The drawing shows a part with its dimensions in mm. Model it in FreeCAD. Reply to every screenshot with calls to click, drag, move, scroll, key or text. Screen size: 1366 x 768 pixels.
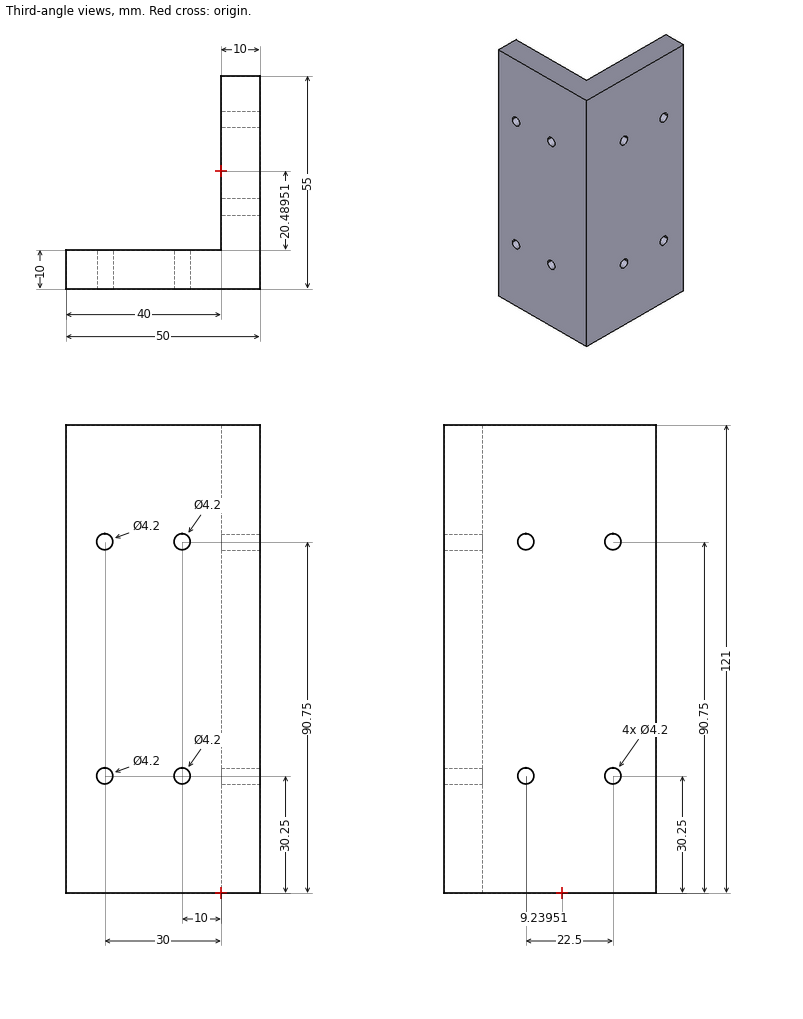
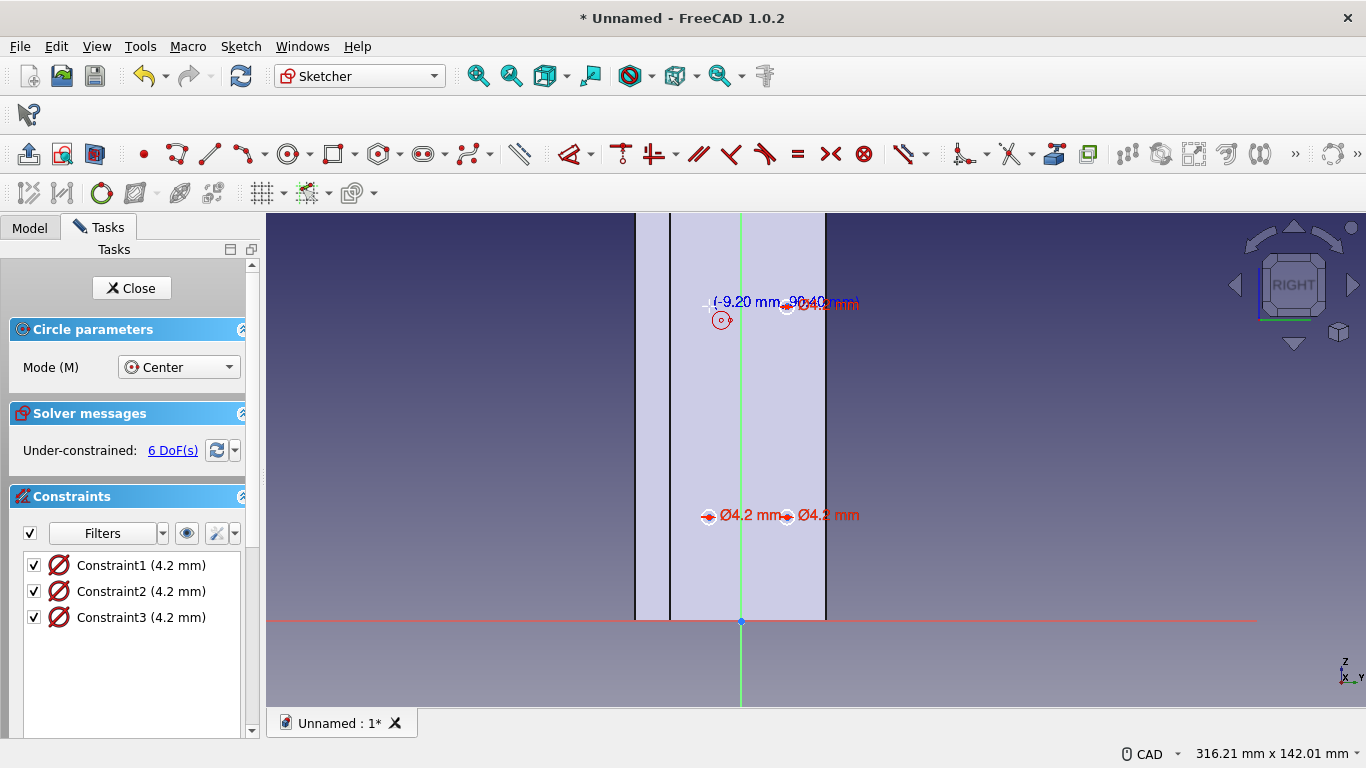
click(709, 306)
move(714, 301)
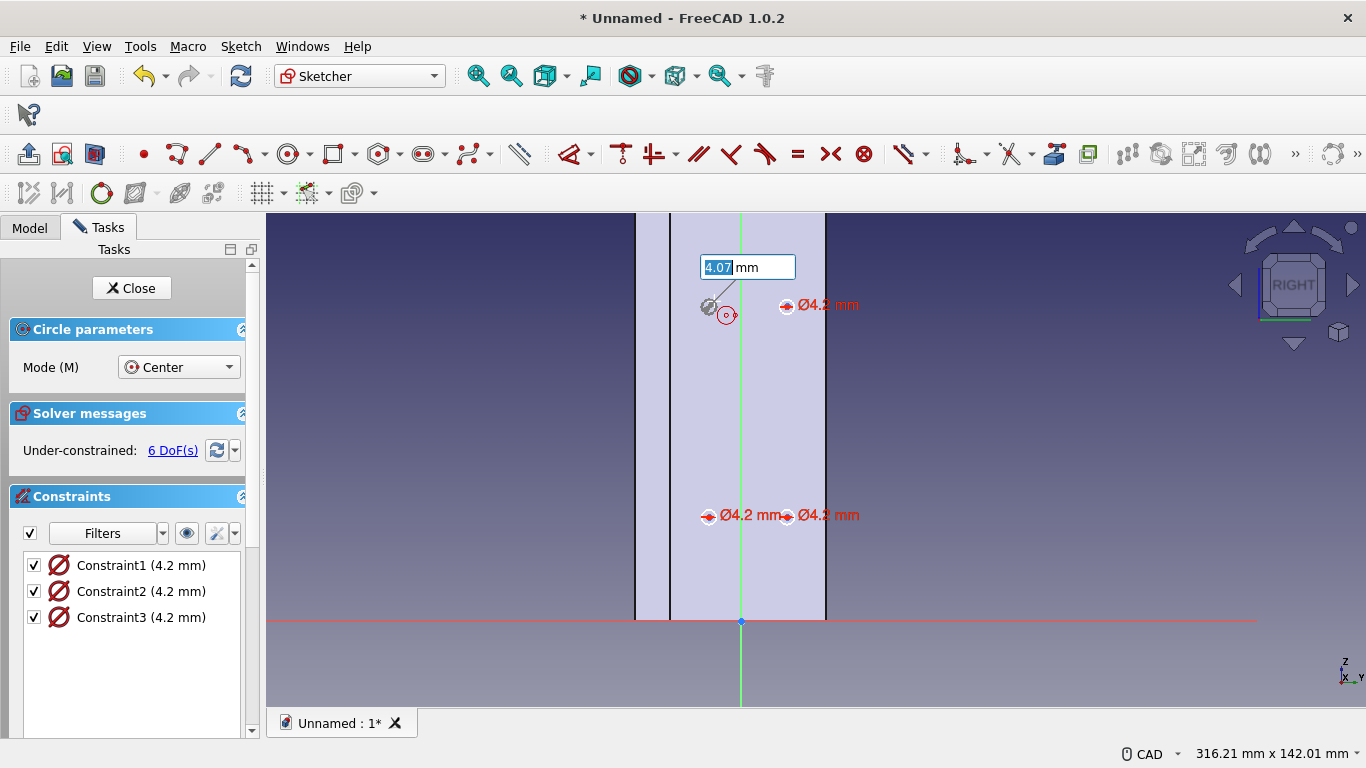
text(4.2)
key(Return)
key(Escape)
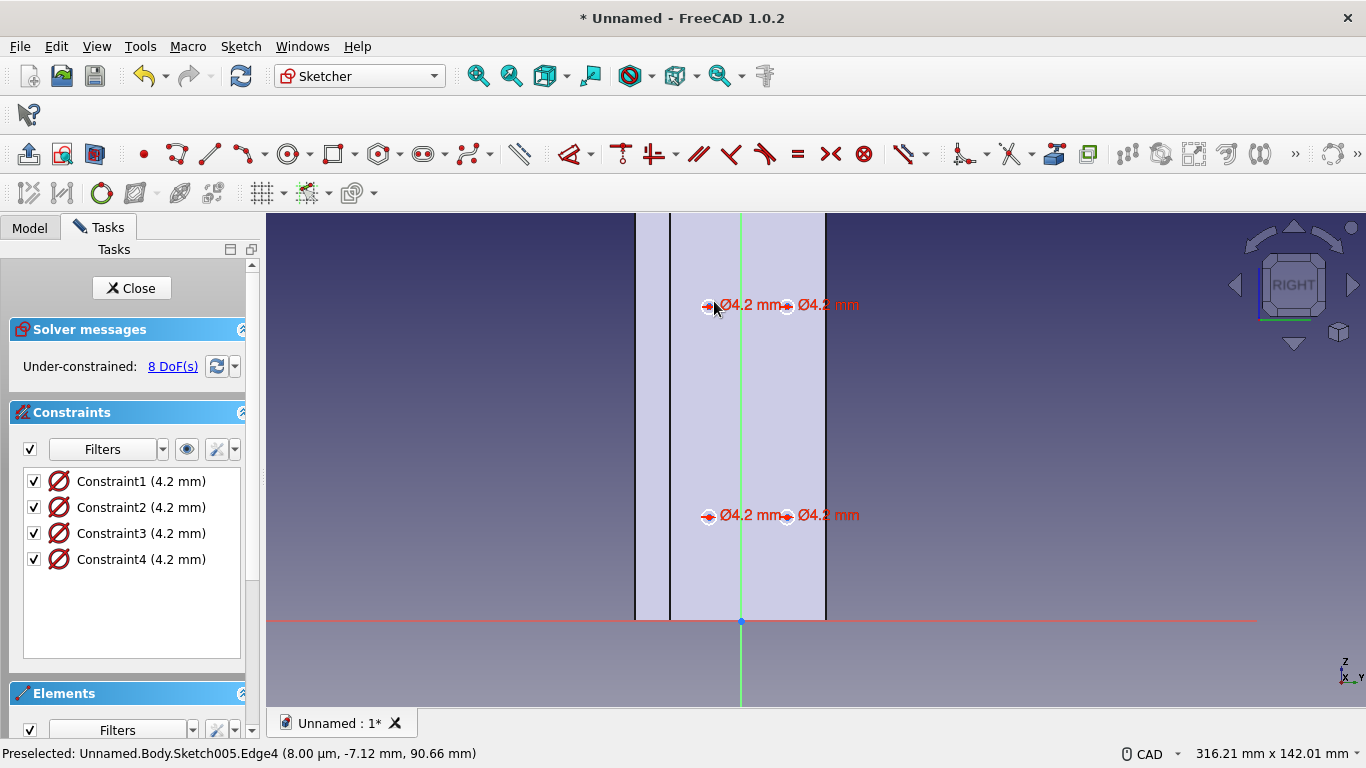
click(787, 517)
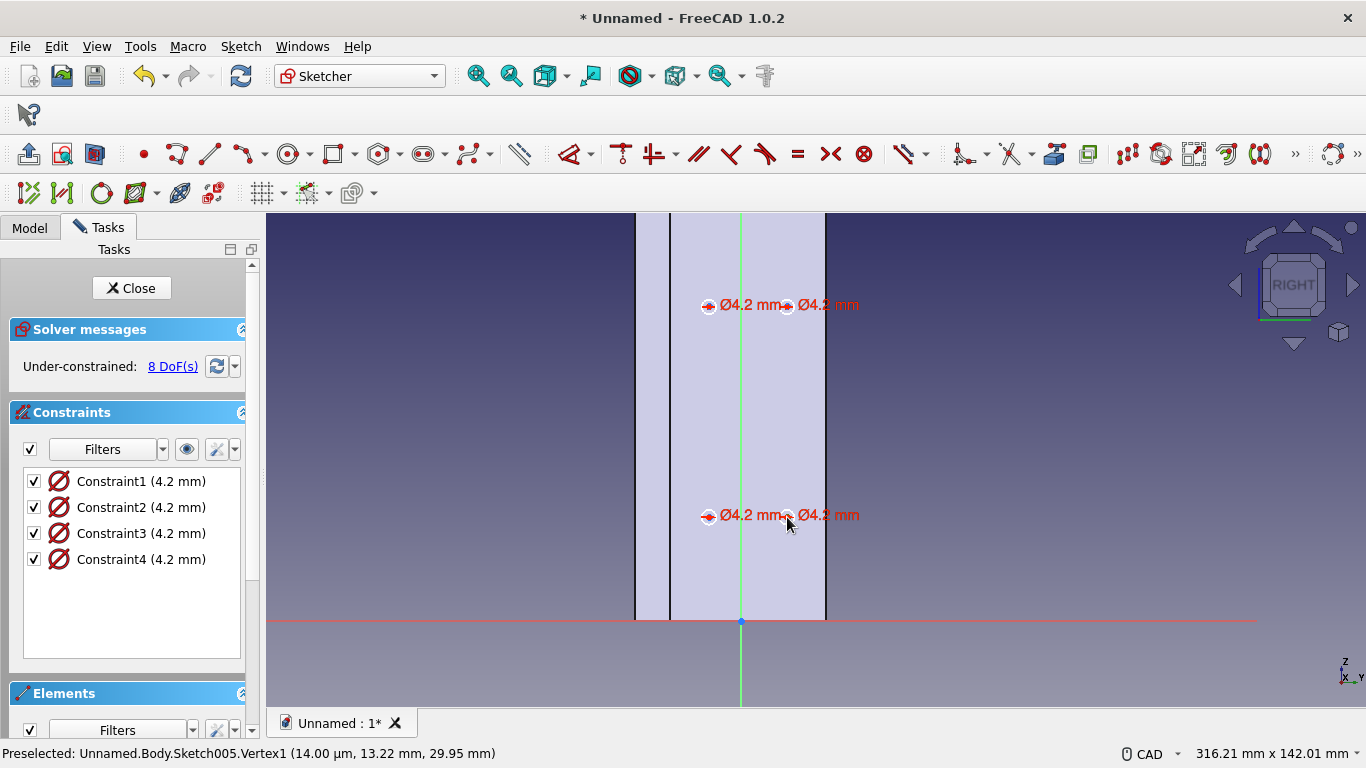
click(709, 517)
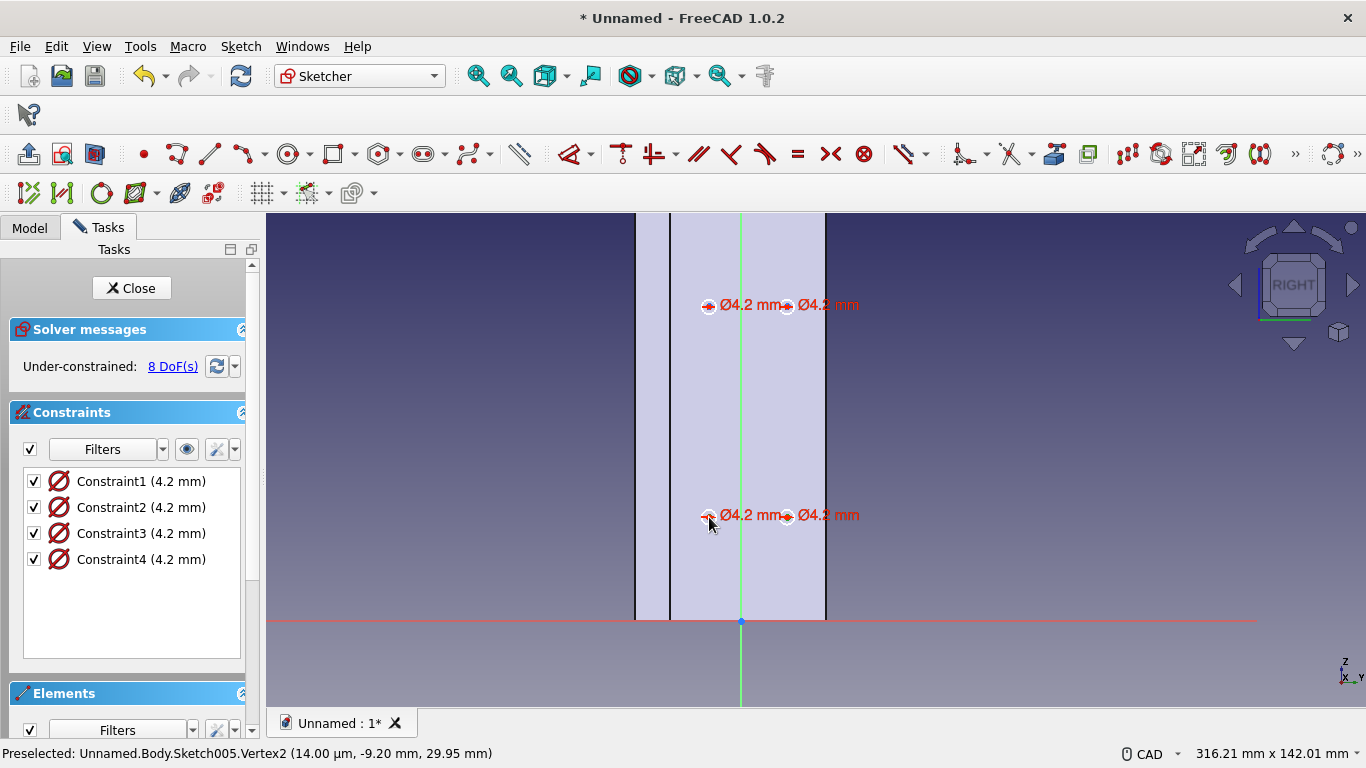
key(h)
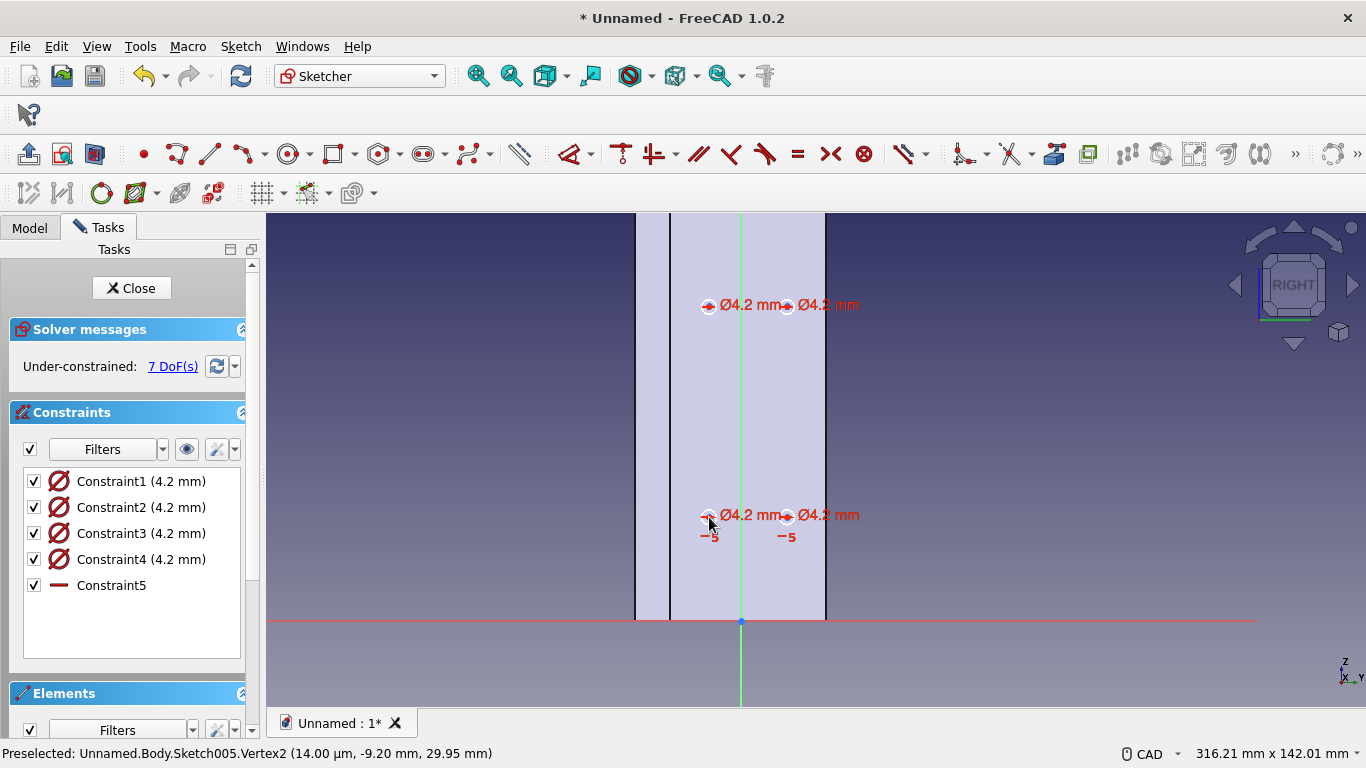
click(787, 517)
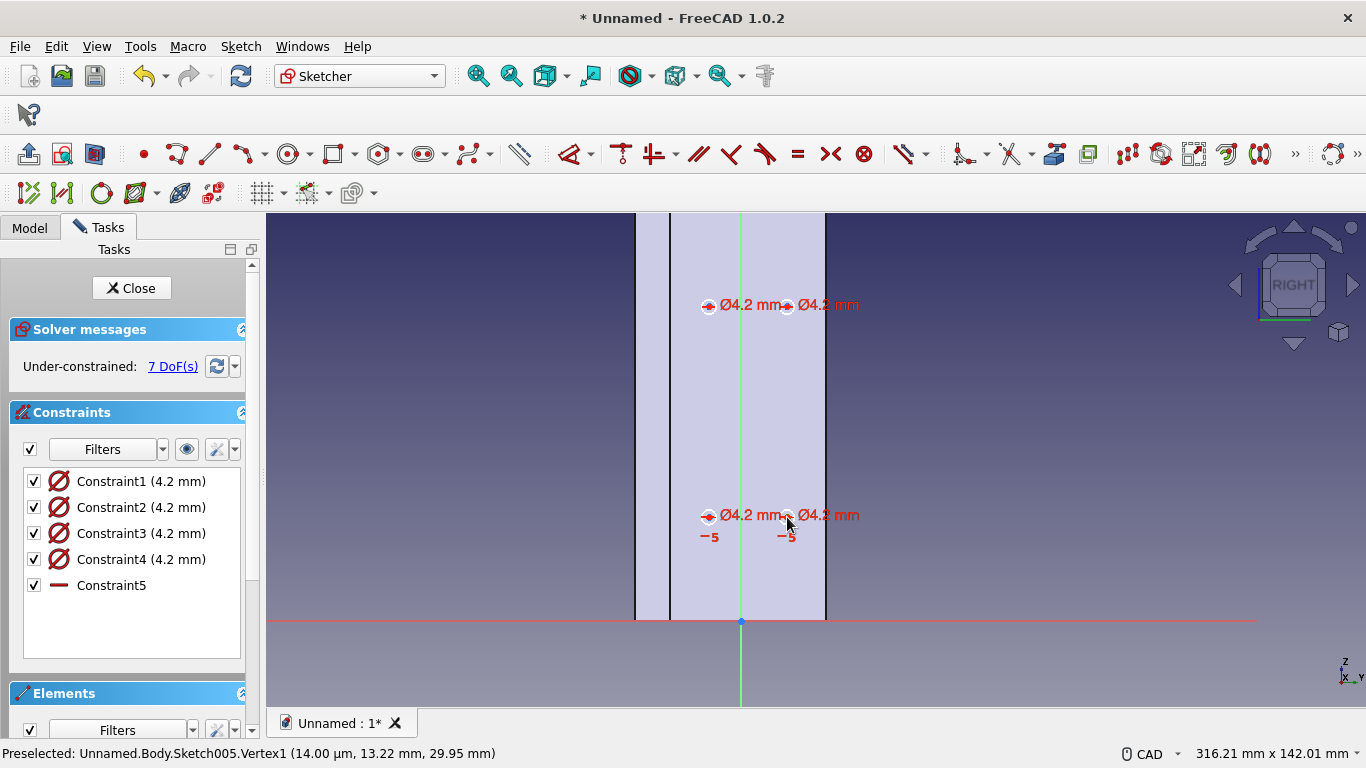
click(787, 307)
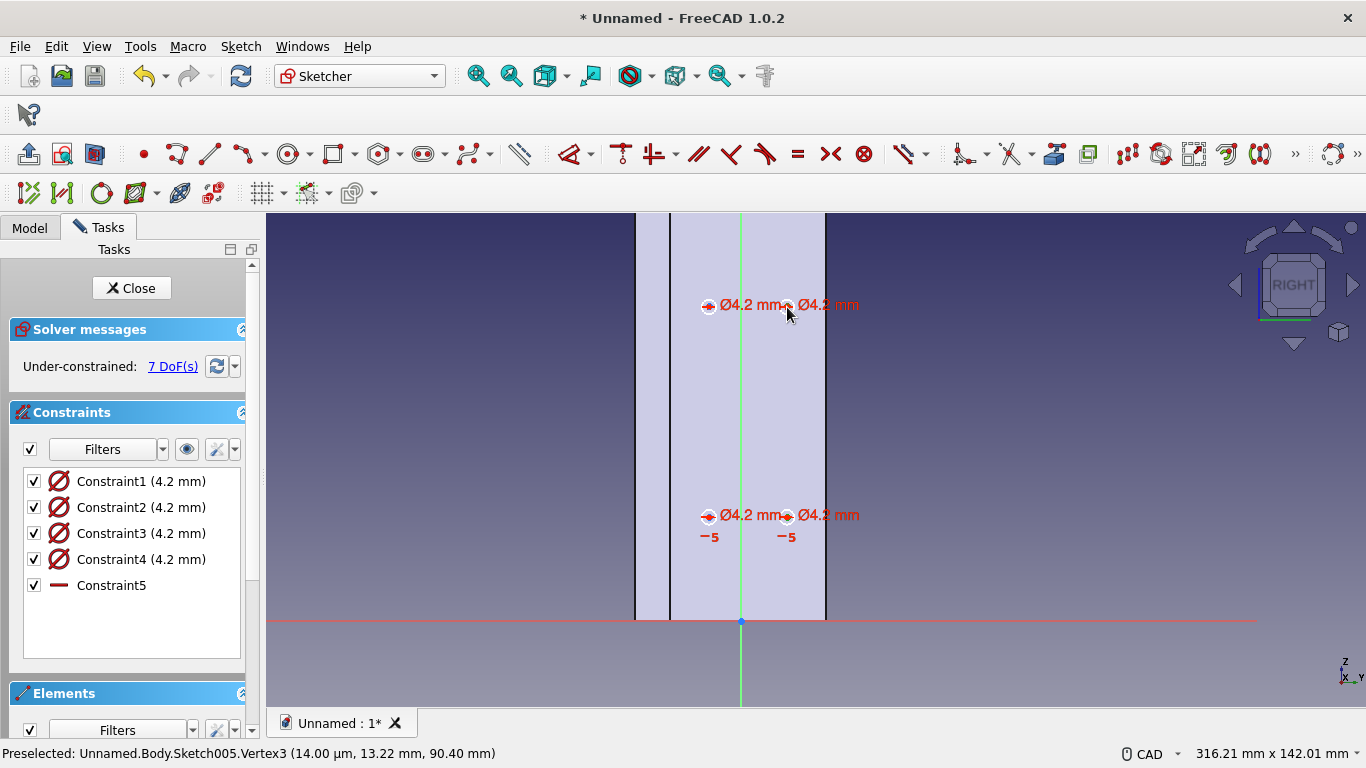
key(v)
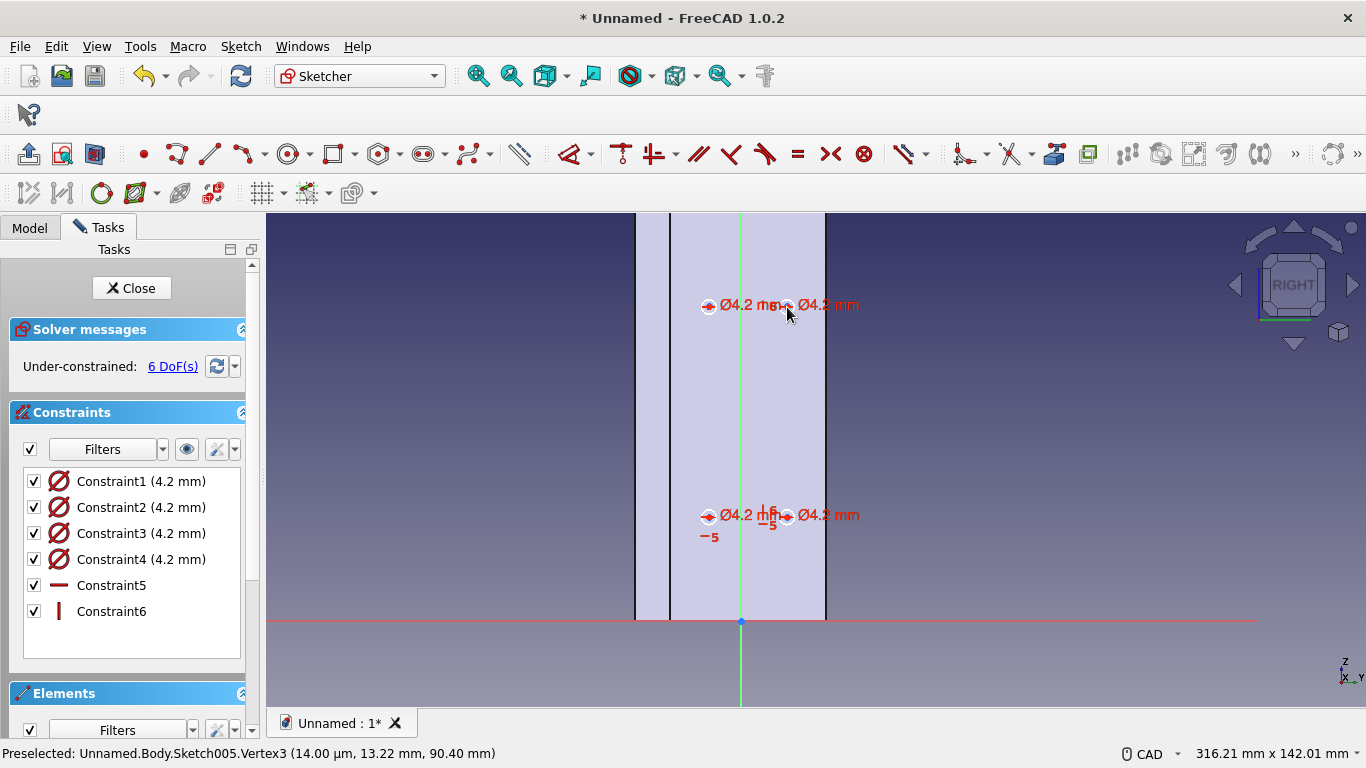
click(709, 517)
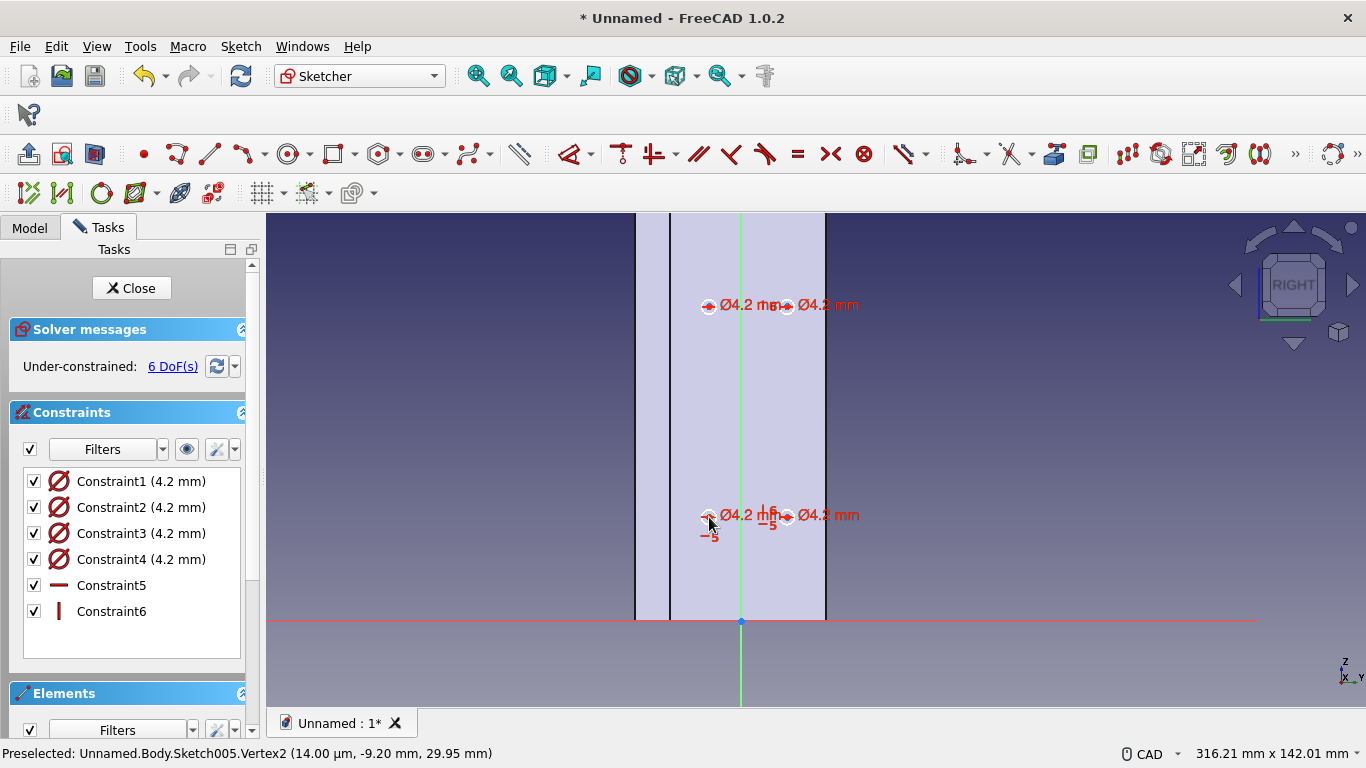
click(709, 307)